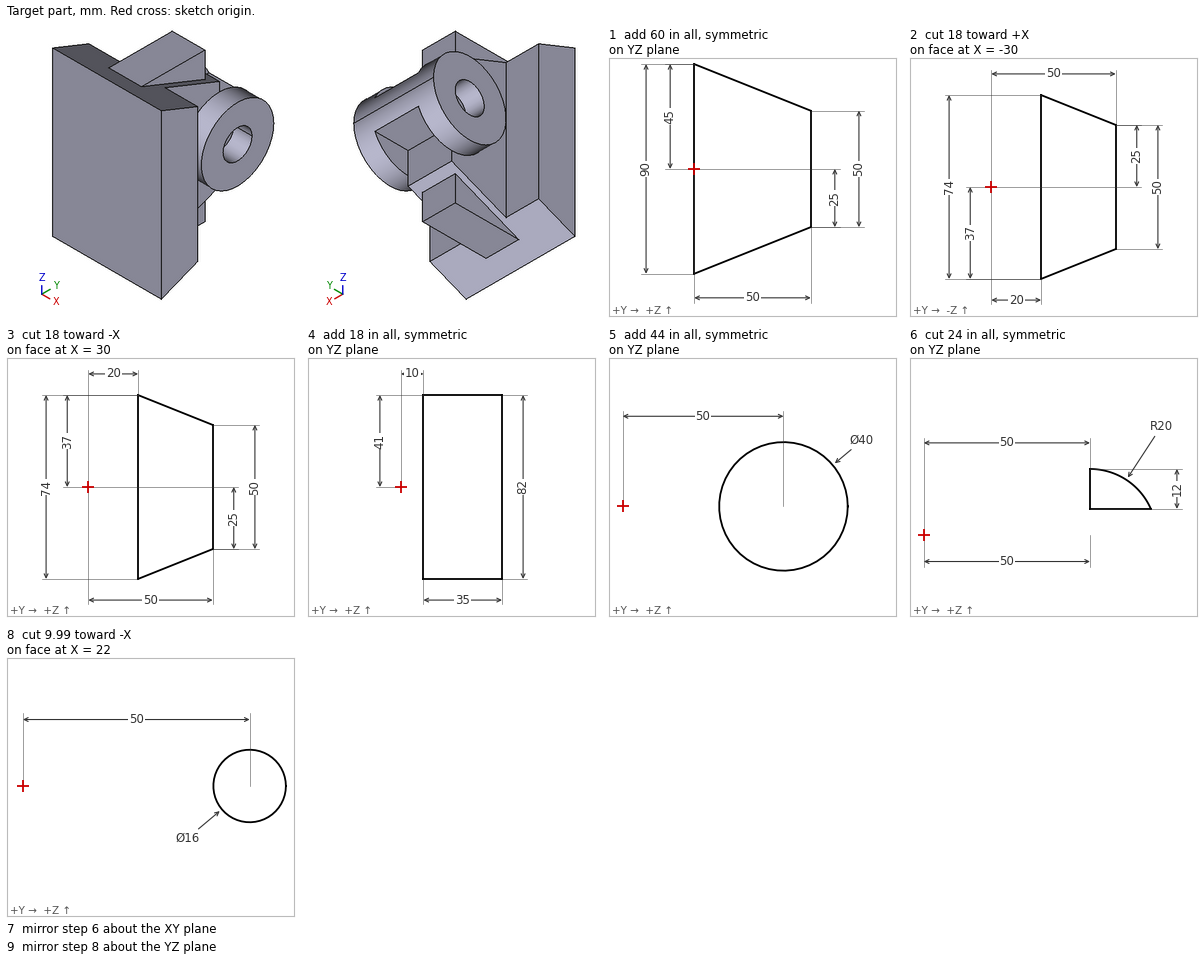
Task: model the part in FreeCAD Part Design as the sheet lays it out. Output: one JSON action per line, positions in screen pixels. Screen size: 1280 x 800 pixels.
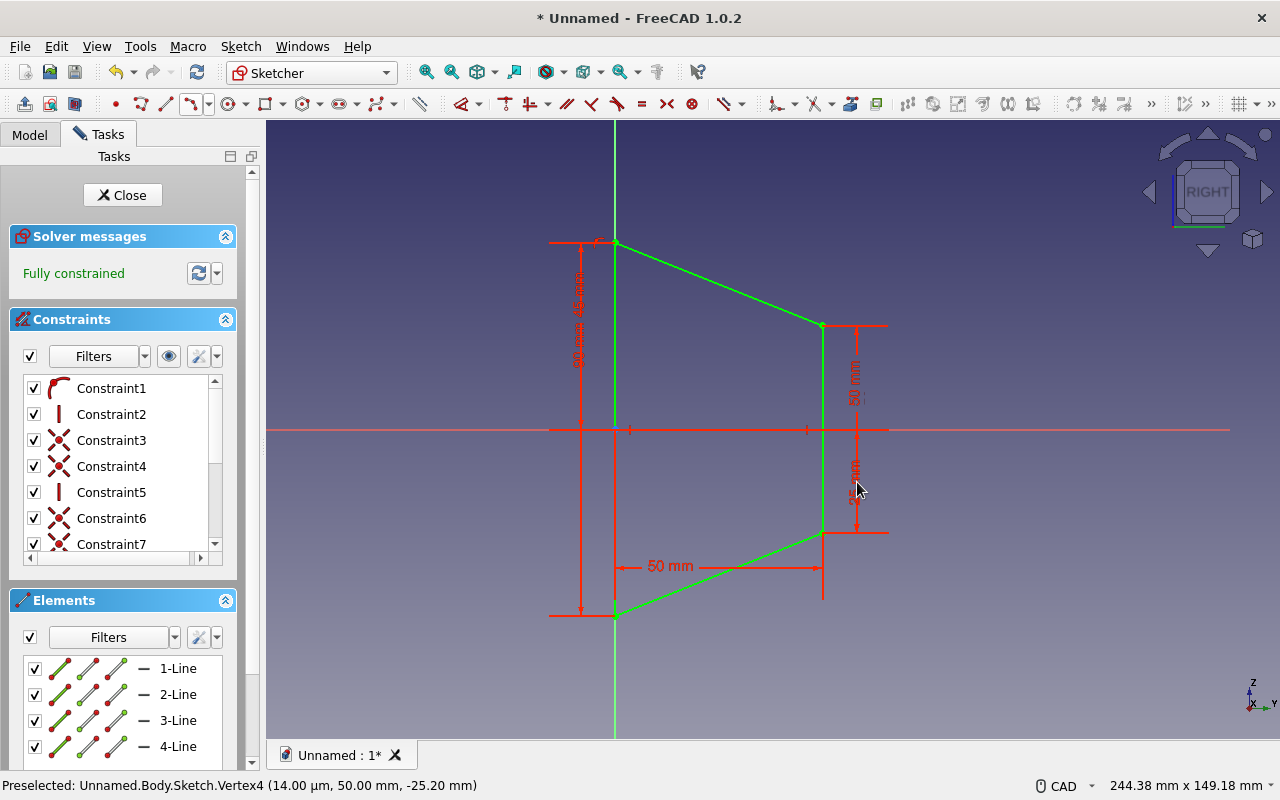
{"action": "left_click", "coordinate": [123, 195]}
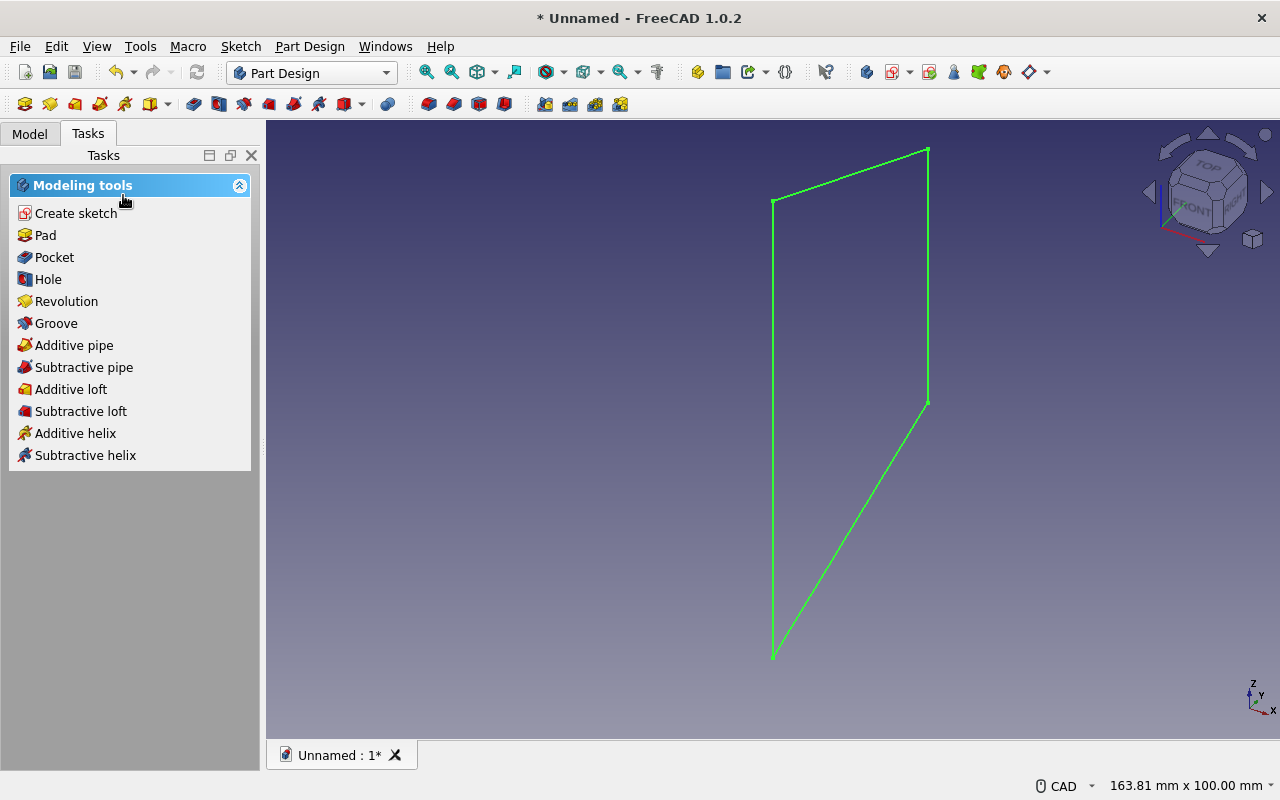
{"action": "left_click", "coordinate": [25, 104]}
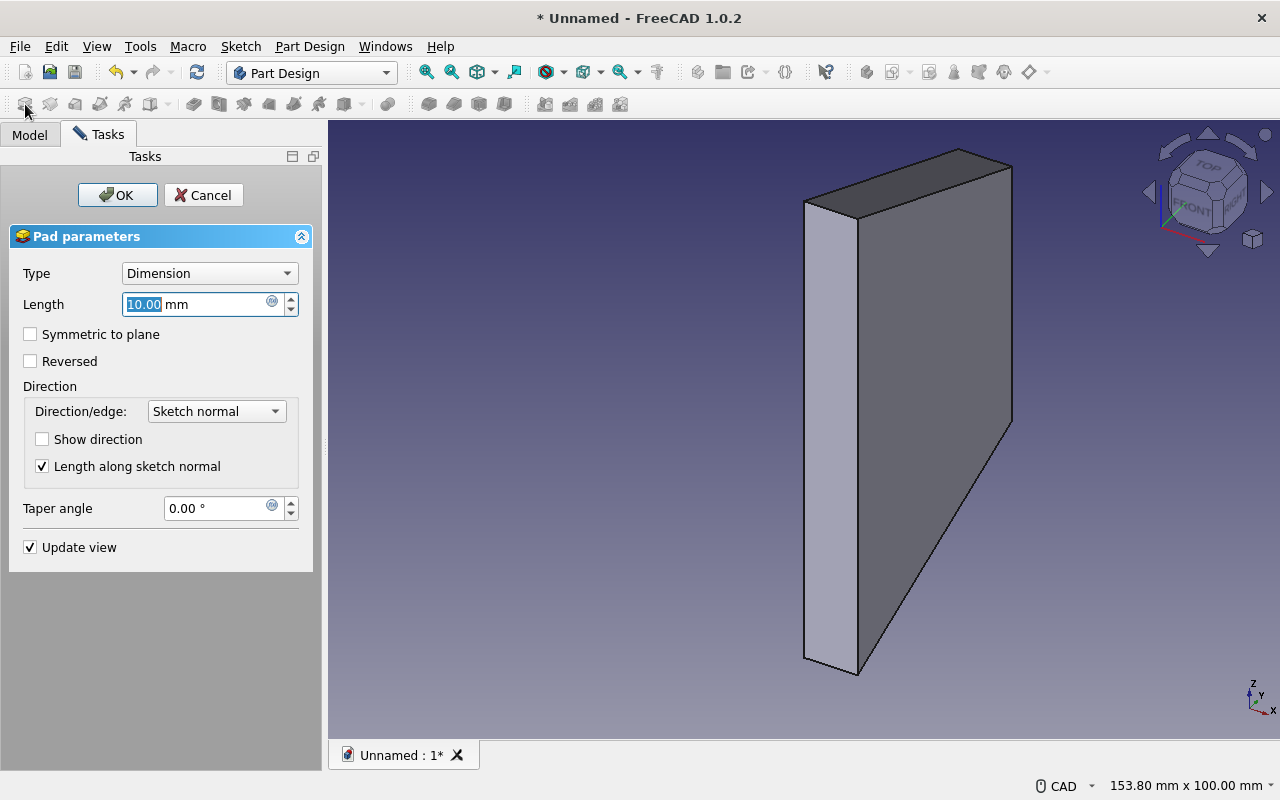
{"action": "type", "text": "60"}
{"action": "key", "text": "Tab"}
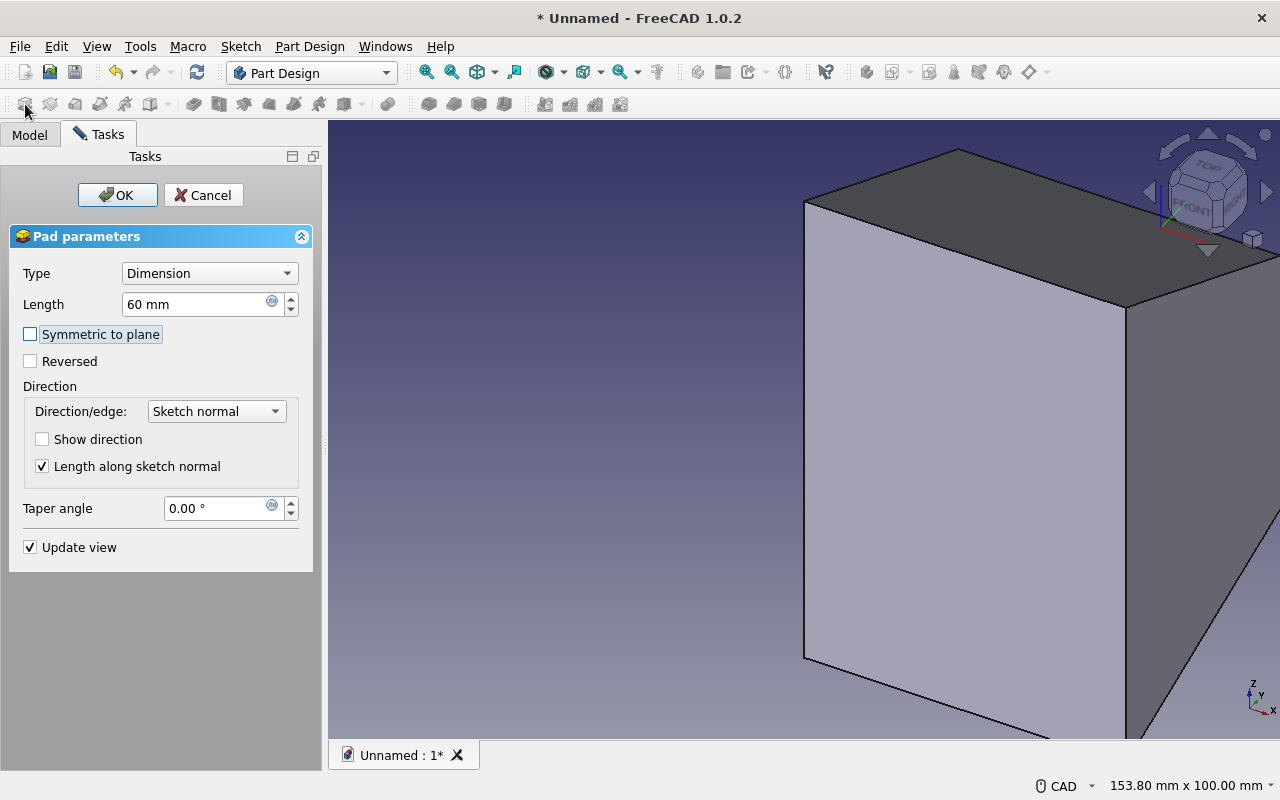
{"action": "left_click", "coordinate": [31, 334]}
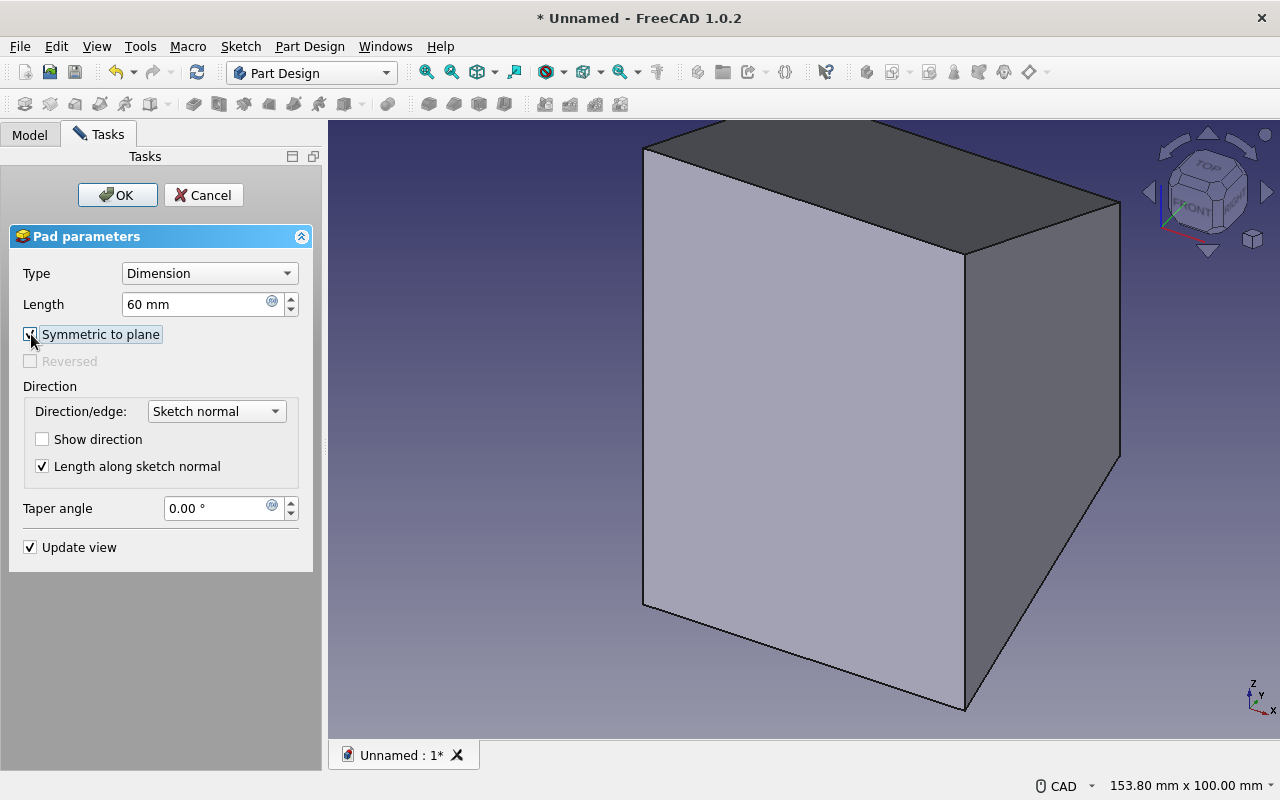
{"action": "left_click", "coordinate": [118, 195]}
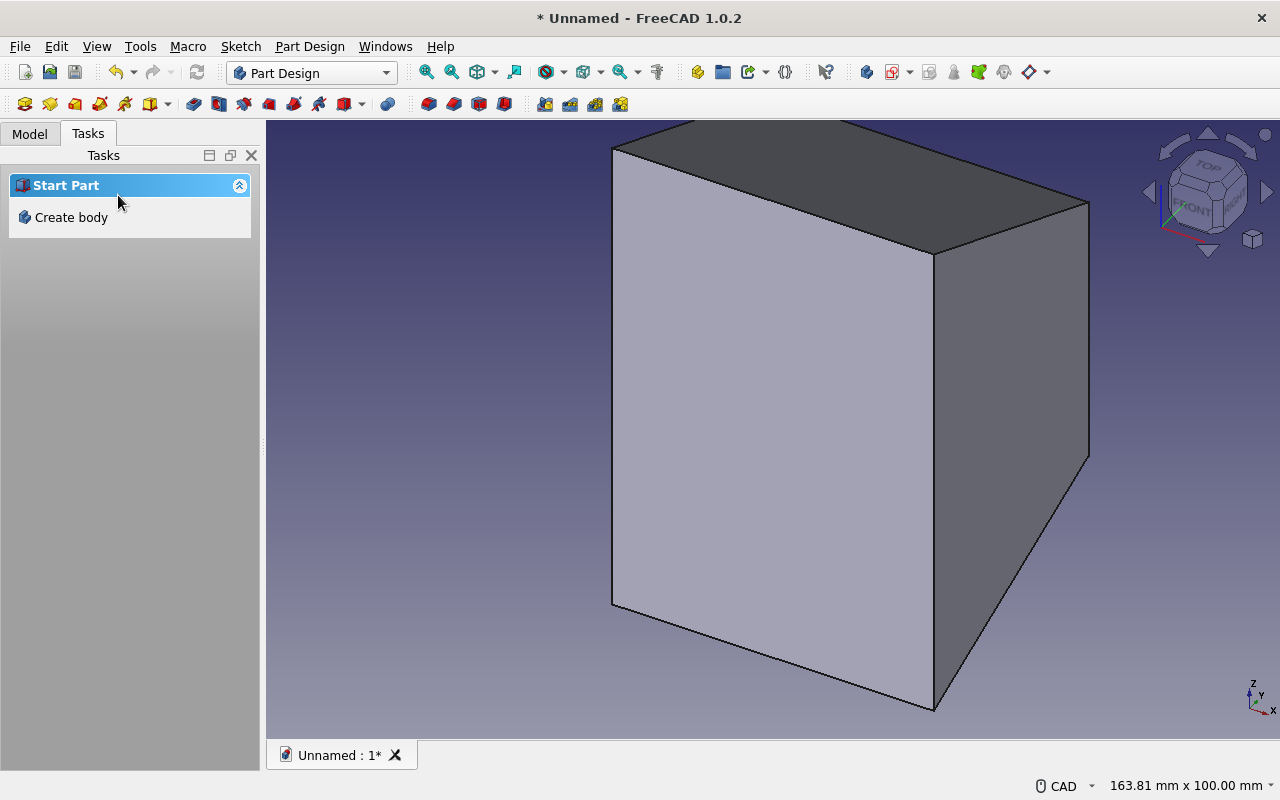
{"action": "left_click", "coordinate": [427, 72]}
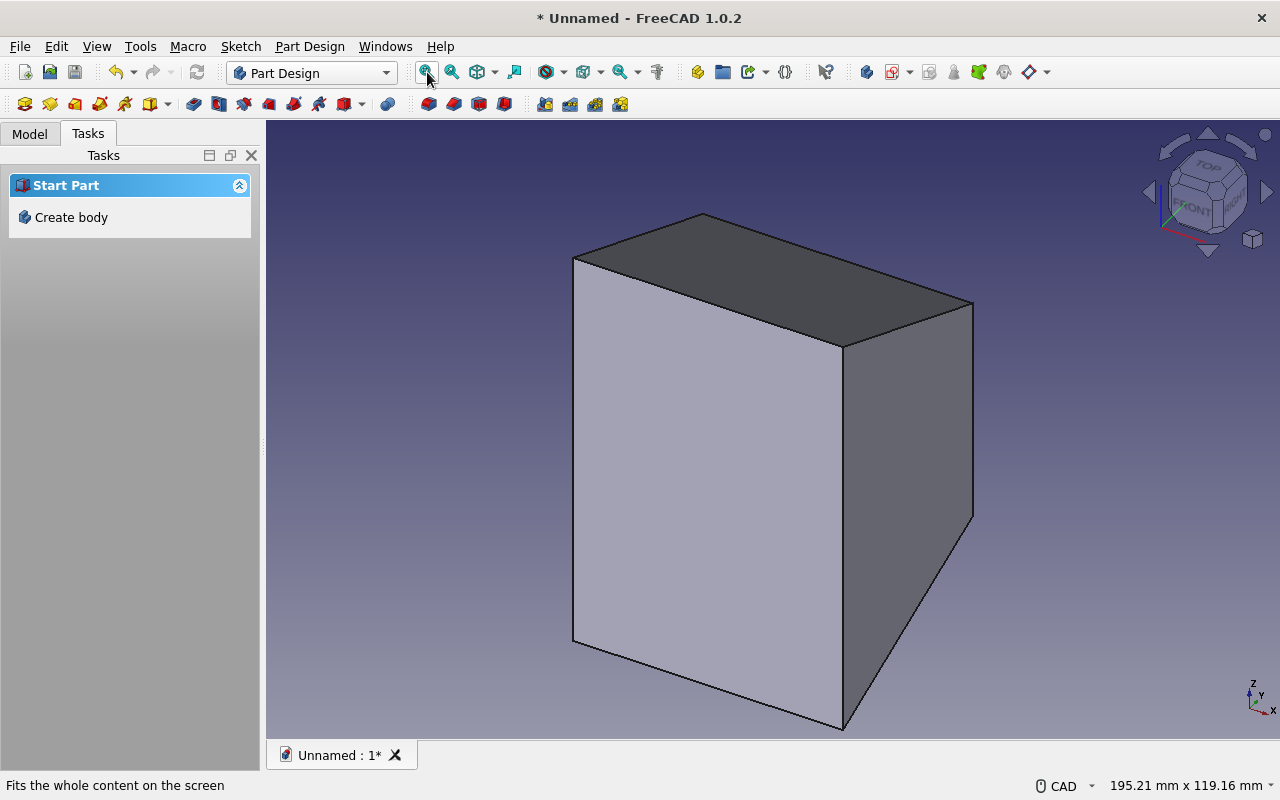
{"action": "key", "text": "6"}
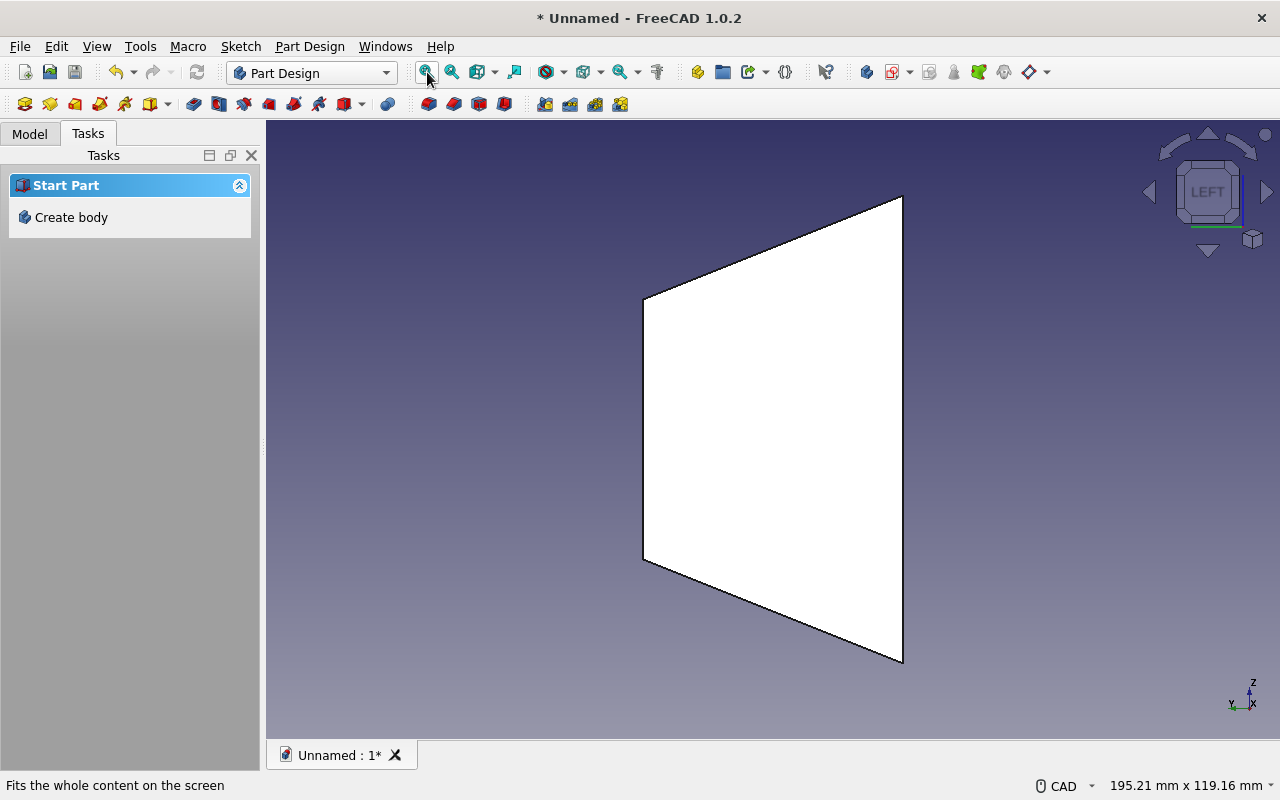
{"action": "left_click", "coordinate": [773, 428]}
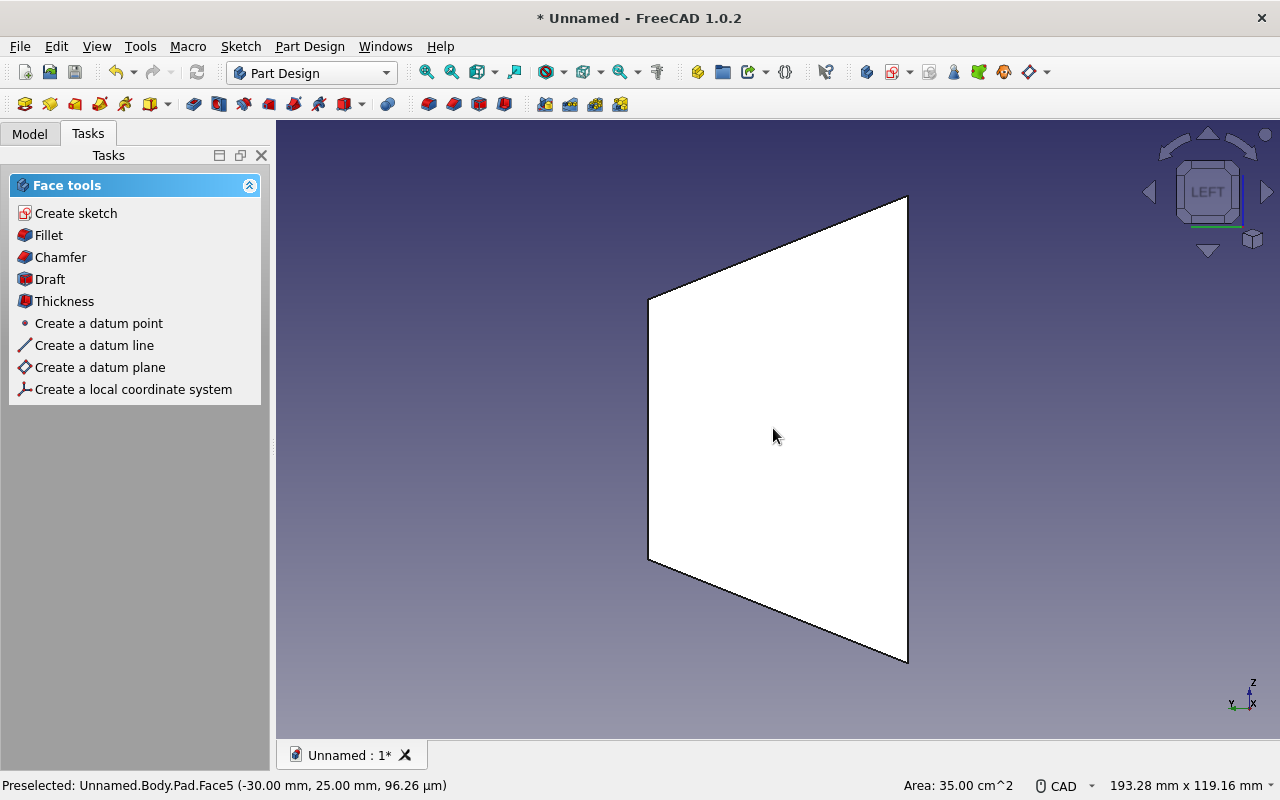
{"action": "left_click", "coordinate": [892, 72]}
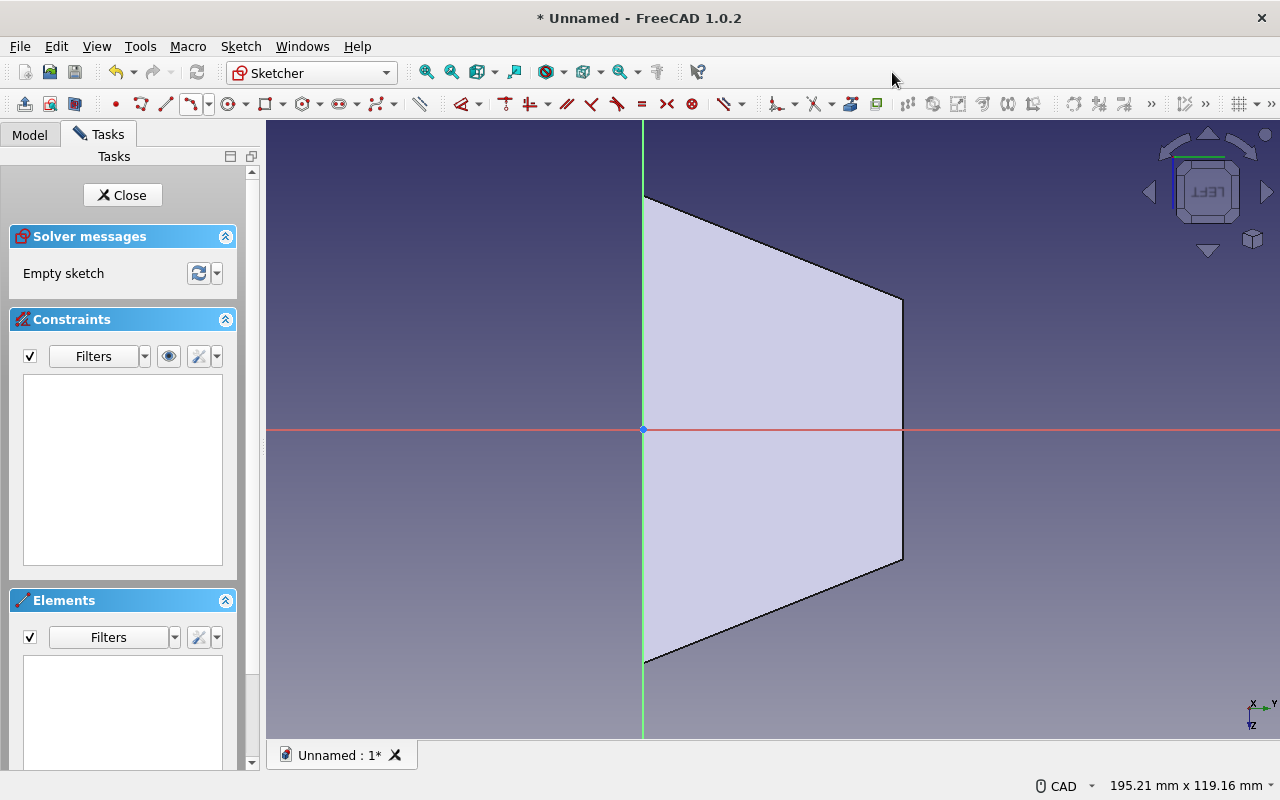
{"action": "key", "text": "g m"}